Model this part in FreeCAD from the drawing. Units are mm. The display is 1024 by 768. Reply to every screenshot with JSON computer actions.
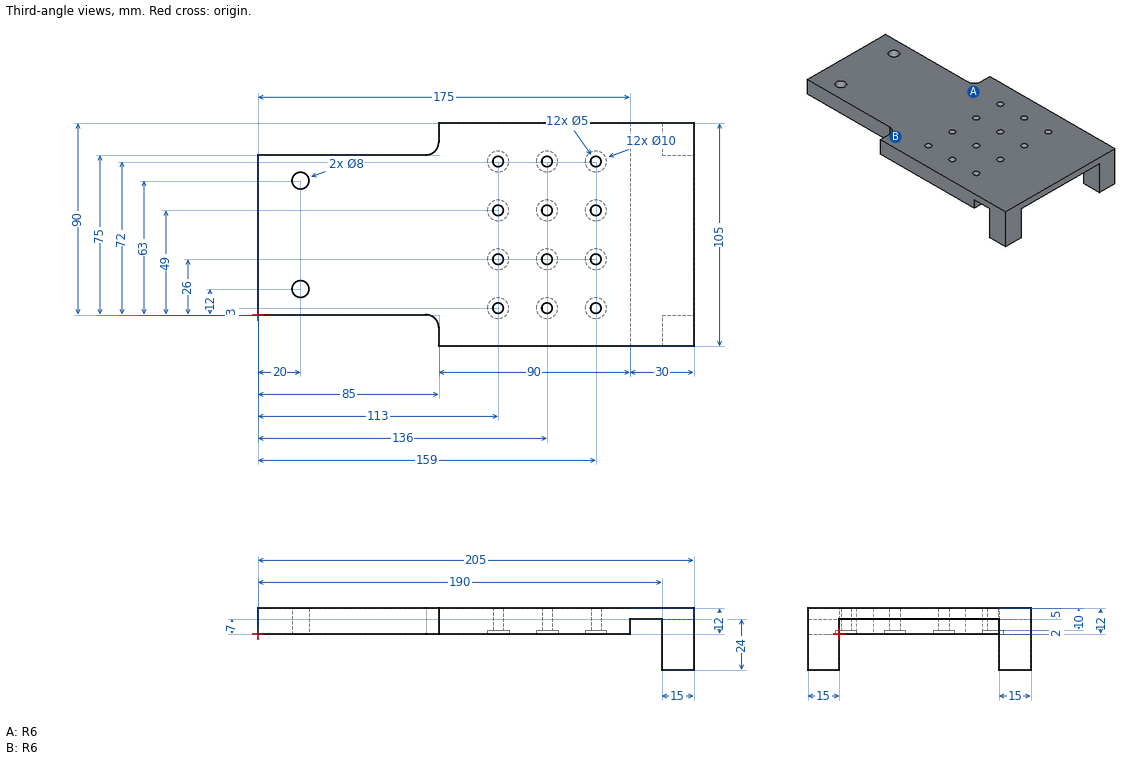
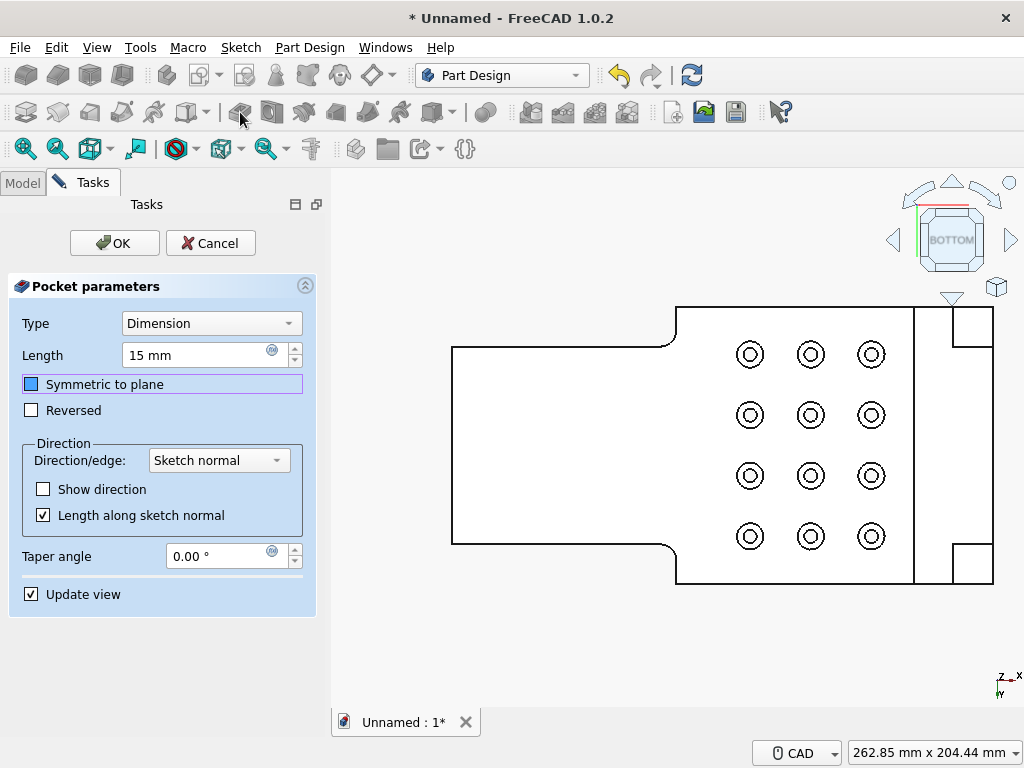
{"action": "left_click", "coordinate": [30, 410]}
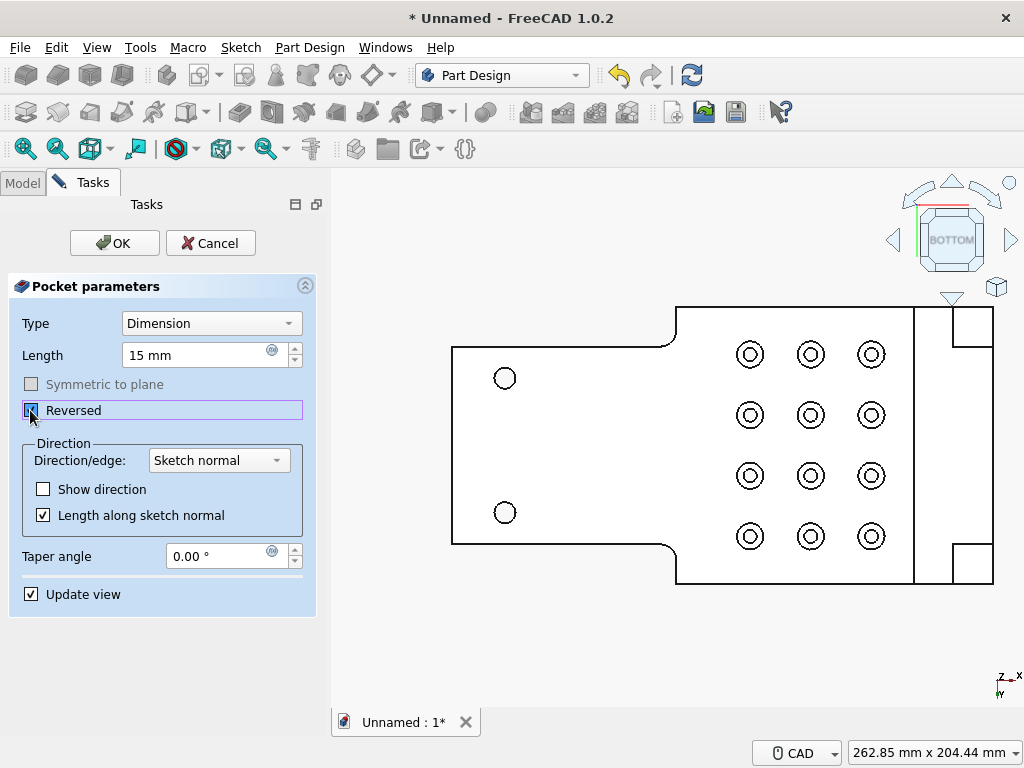
{"action": "left_click", "coordinate": [115, 243]}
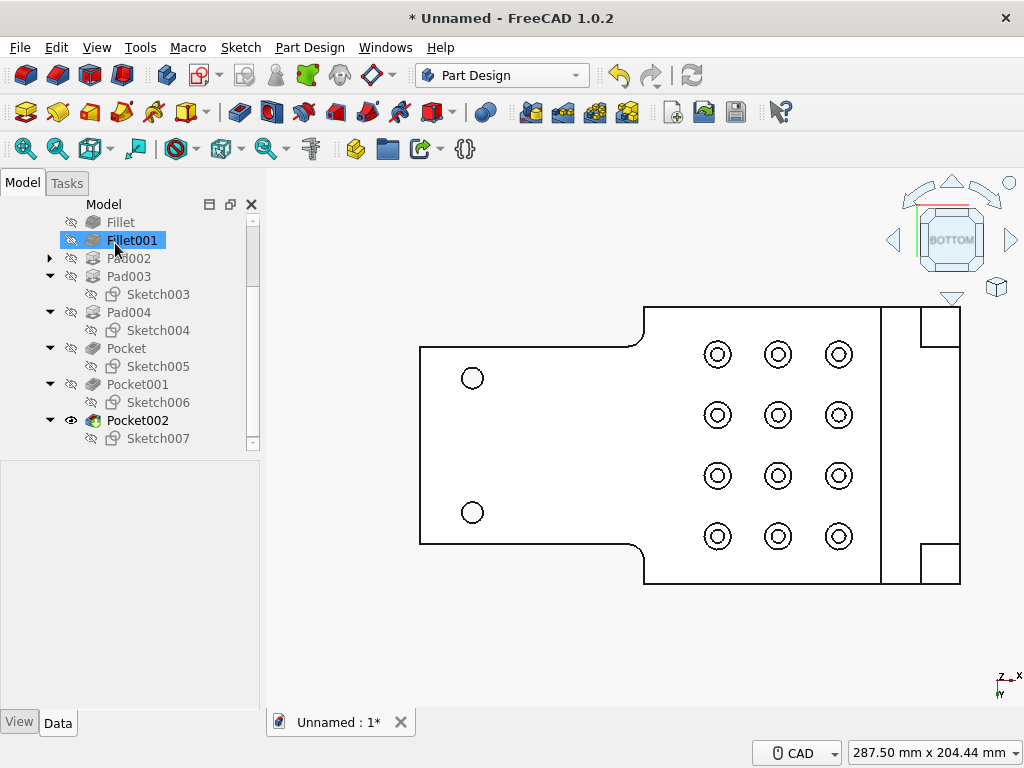
{"action": "key", "text": "0"}